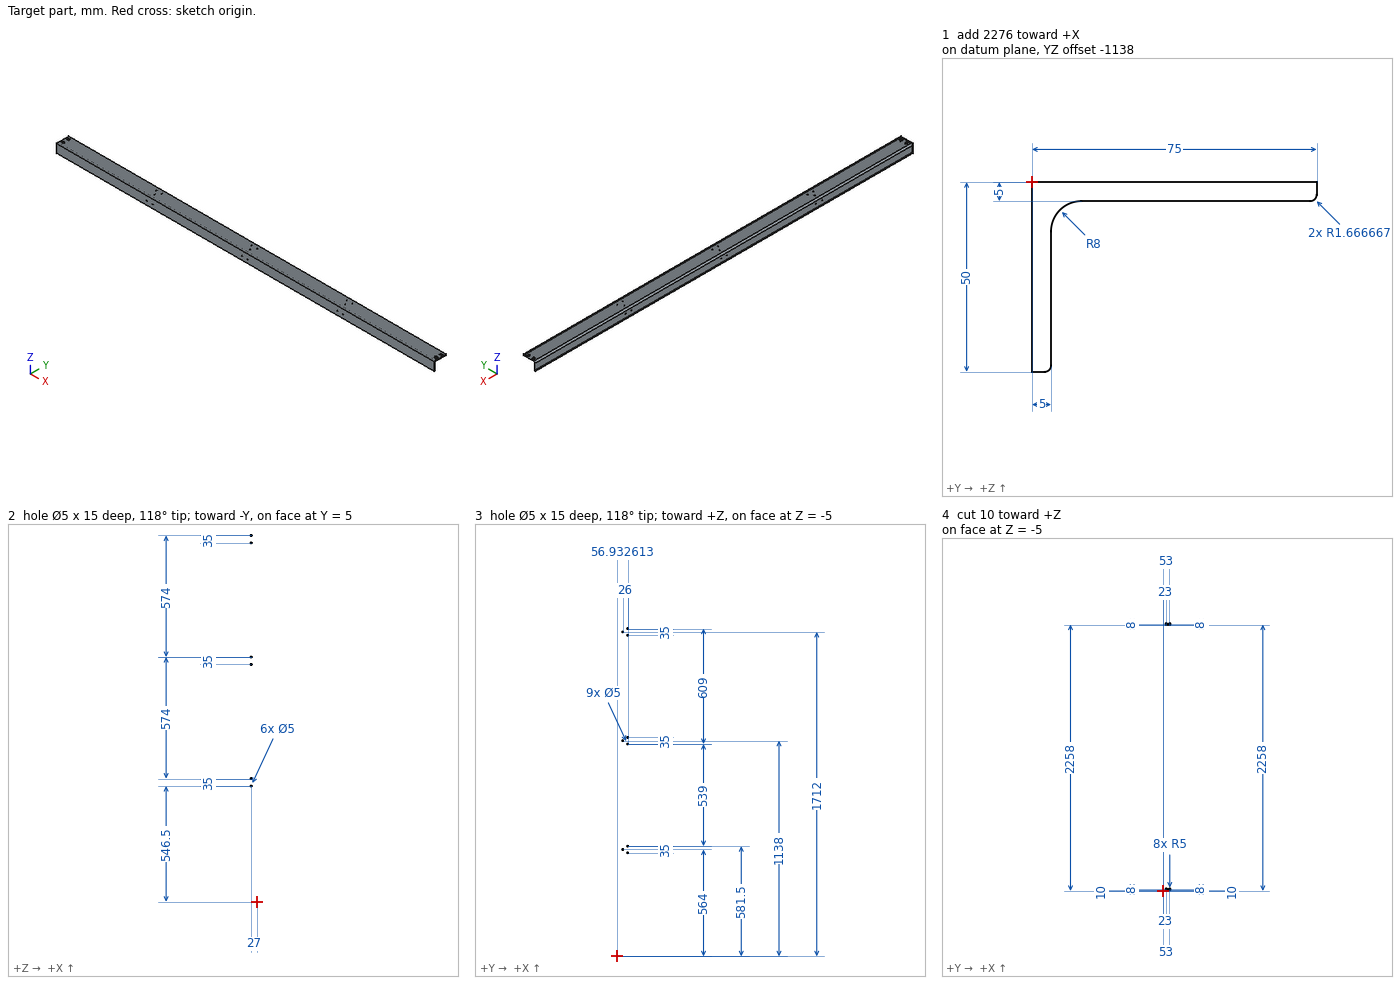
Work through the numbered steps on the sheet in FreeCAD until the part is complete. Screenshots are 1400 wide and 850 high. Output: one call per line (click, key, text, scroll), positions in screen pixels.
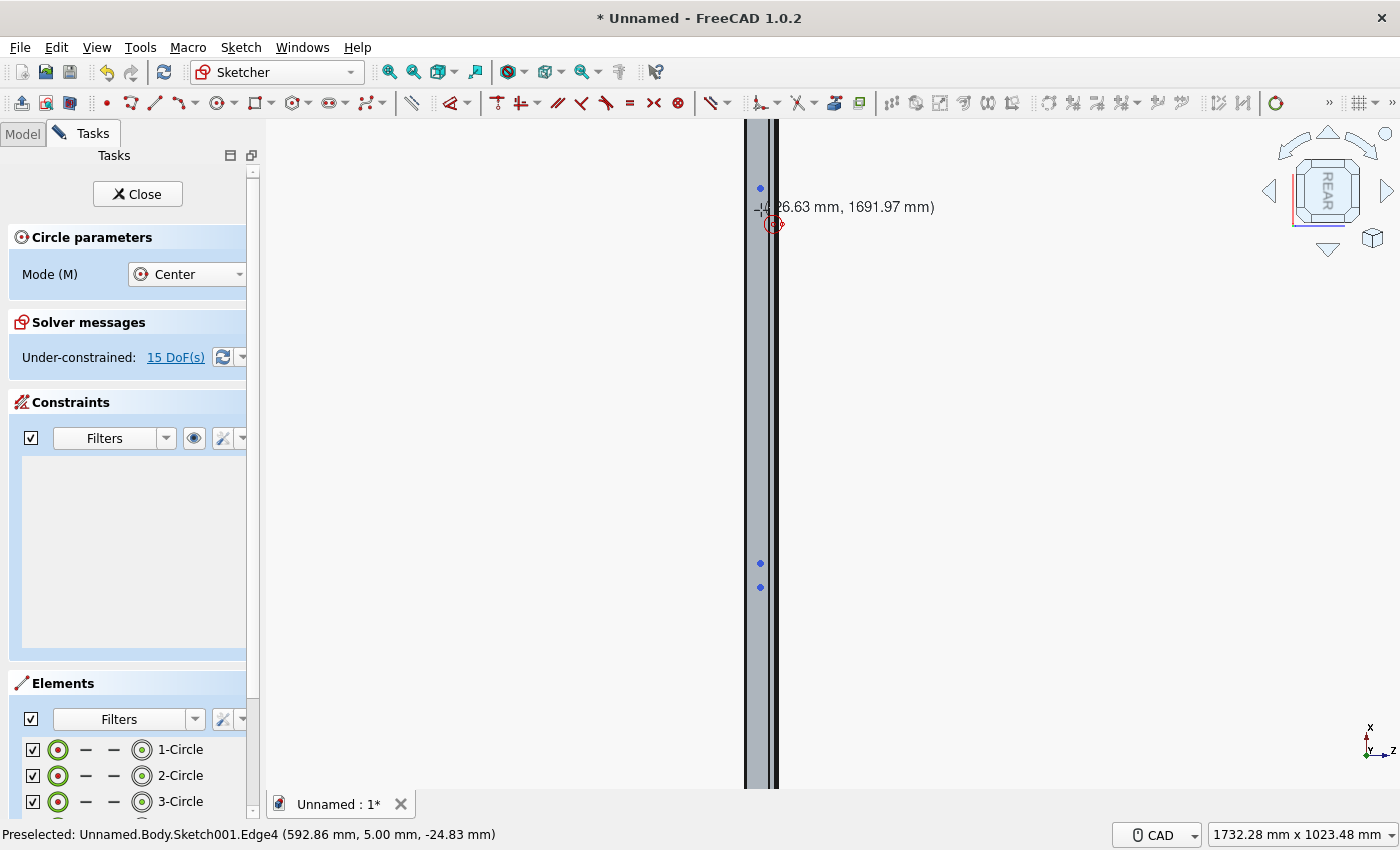
click(760, 210)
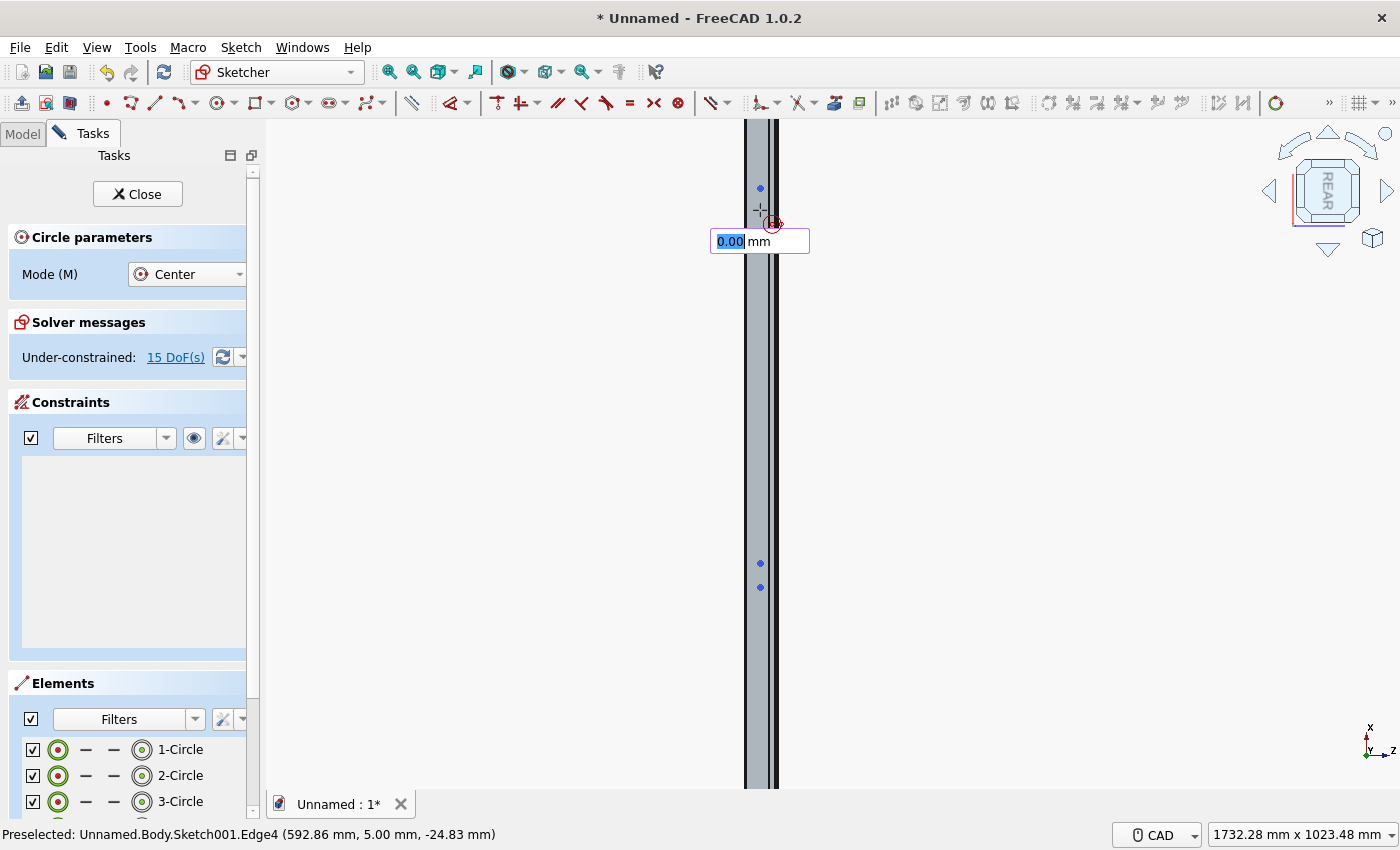
scroll(761, 209, up, 12)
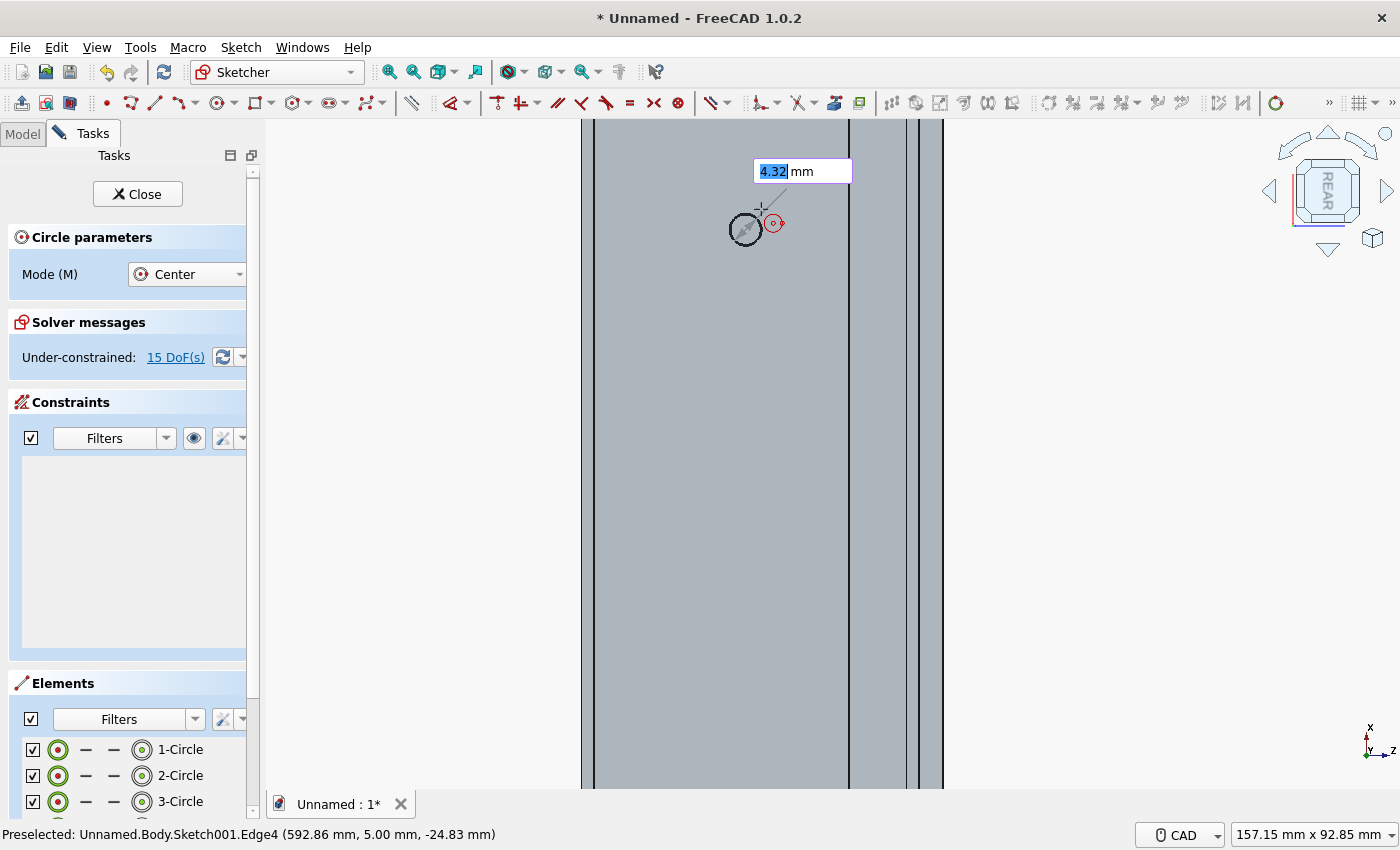
click(761, 210)
key(Escape)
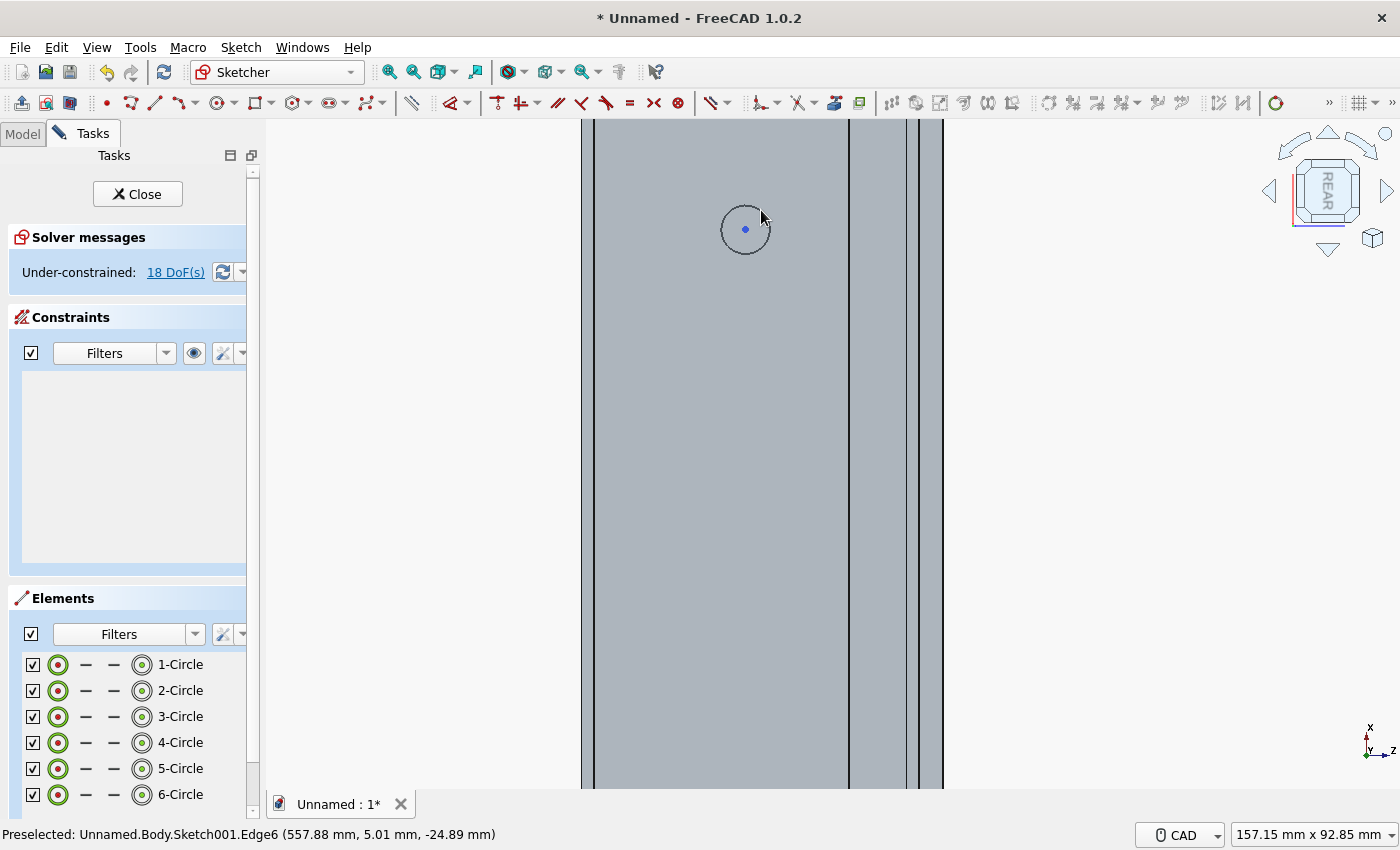
scroll(761, 210, down, 16)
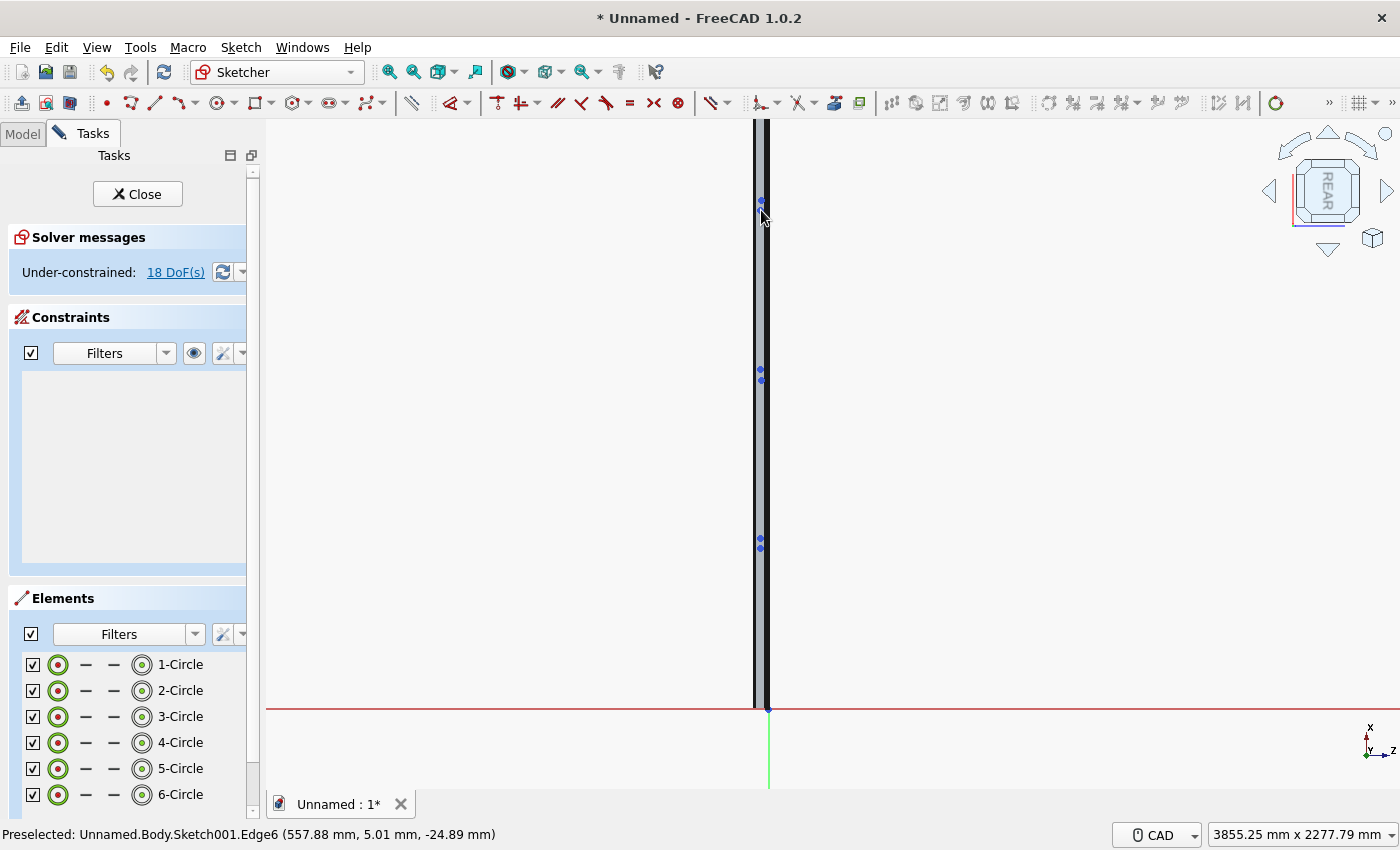
scroll(762, 548, up, 13)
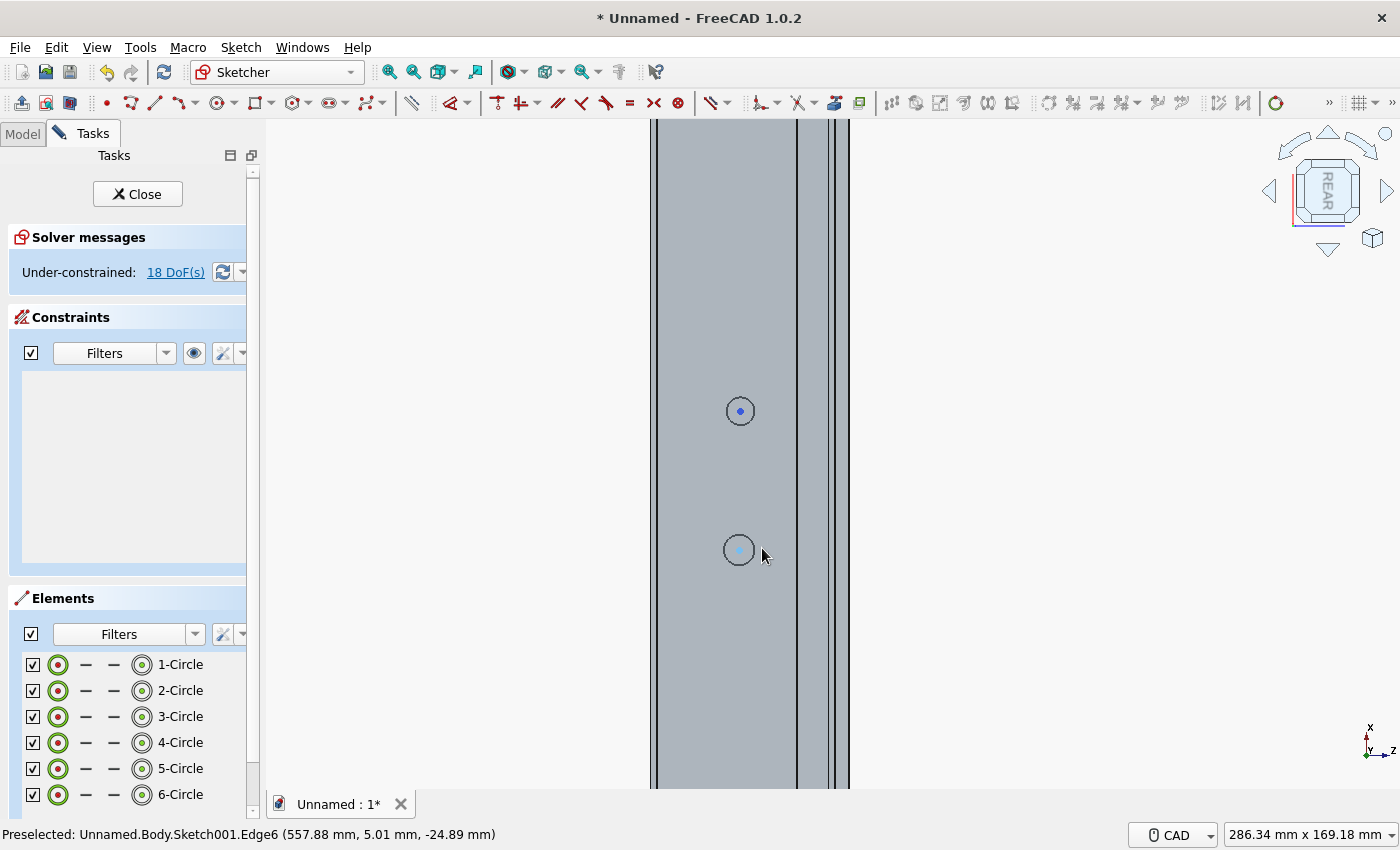
click(750, 539)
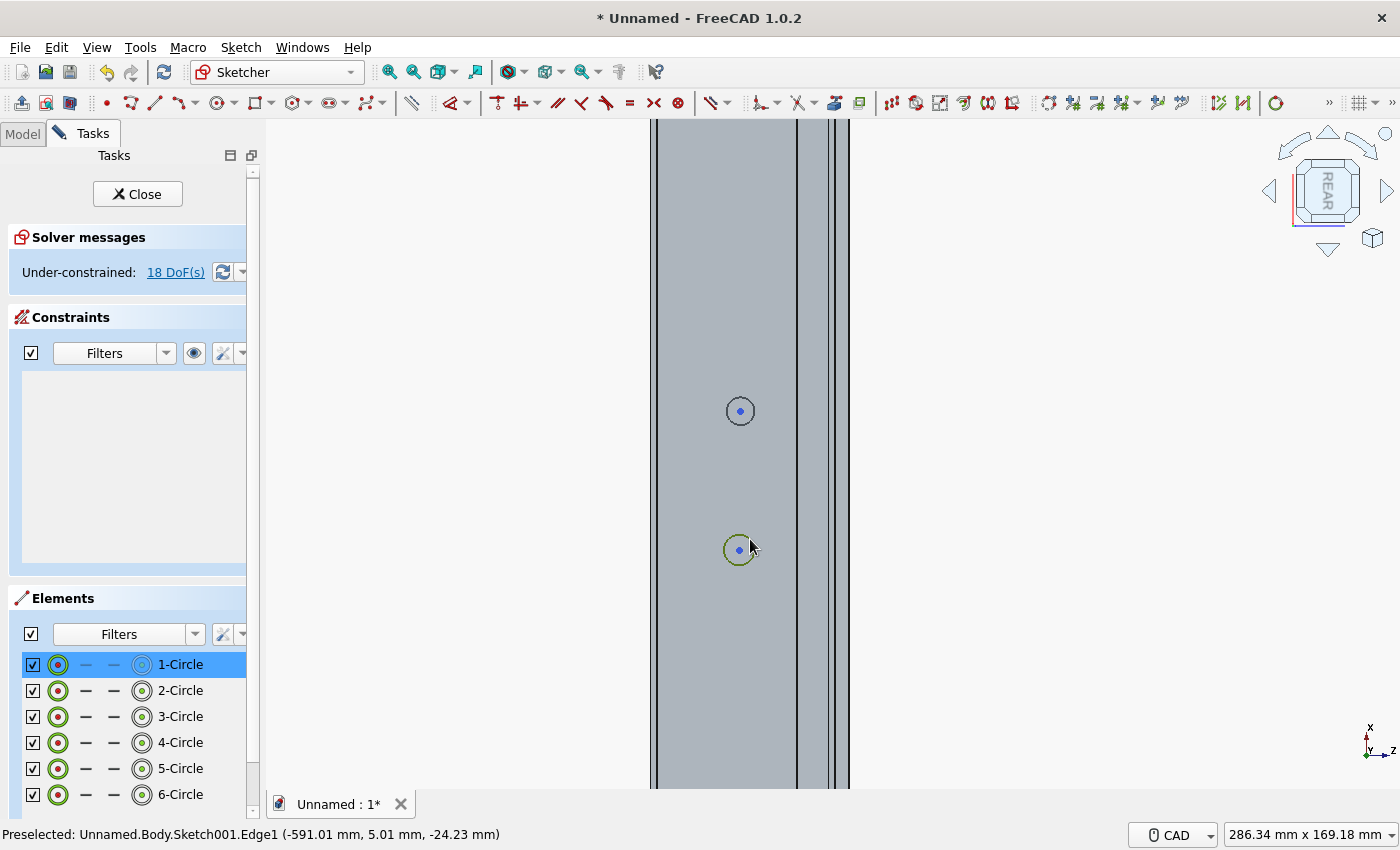
click(750, 401)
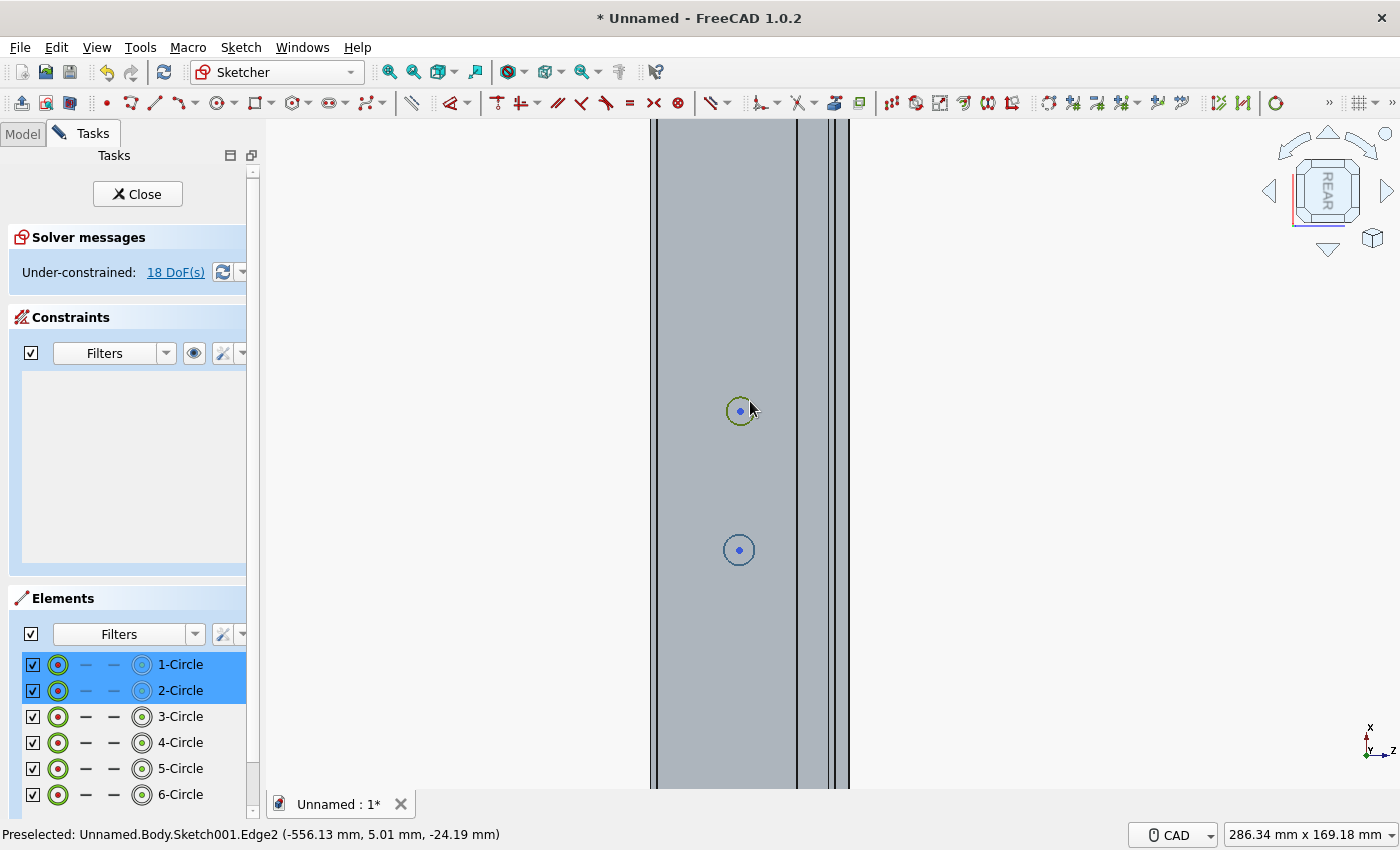
scroll(763, 530, down, 14)